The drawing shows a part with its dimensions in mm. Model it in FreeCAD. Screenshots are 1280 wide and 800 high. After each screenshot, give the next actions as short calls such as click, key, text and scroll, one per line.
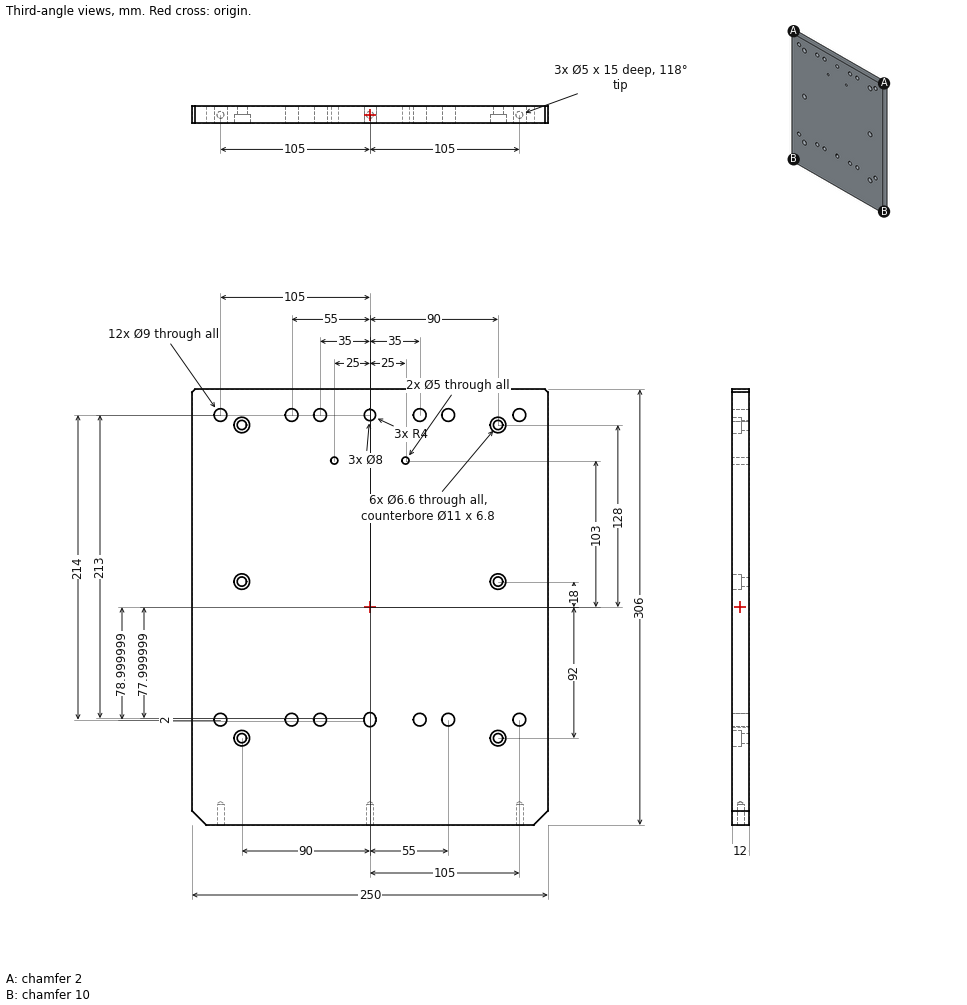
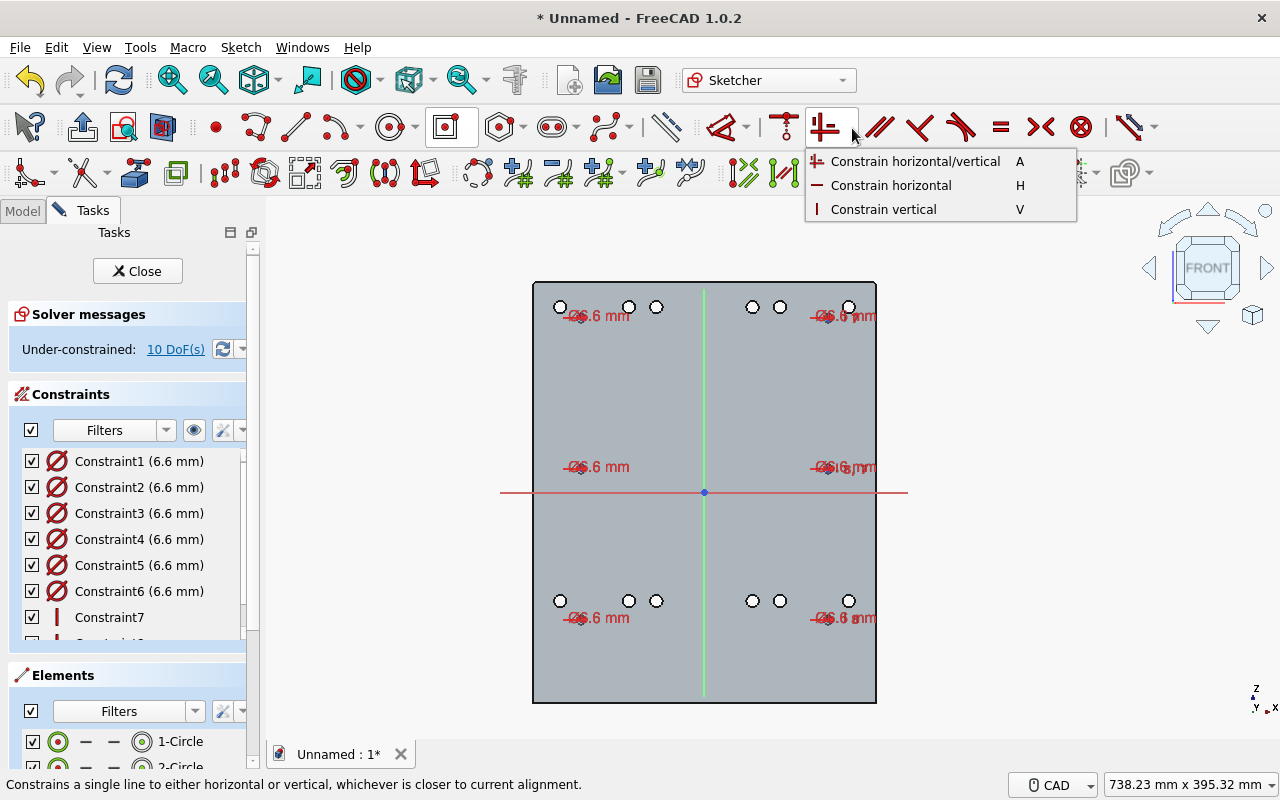
click(941, 185)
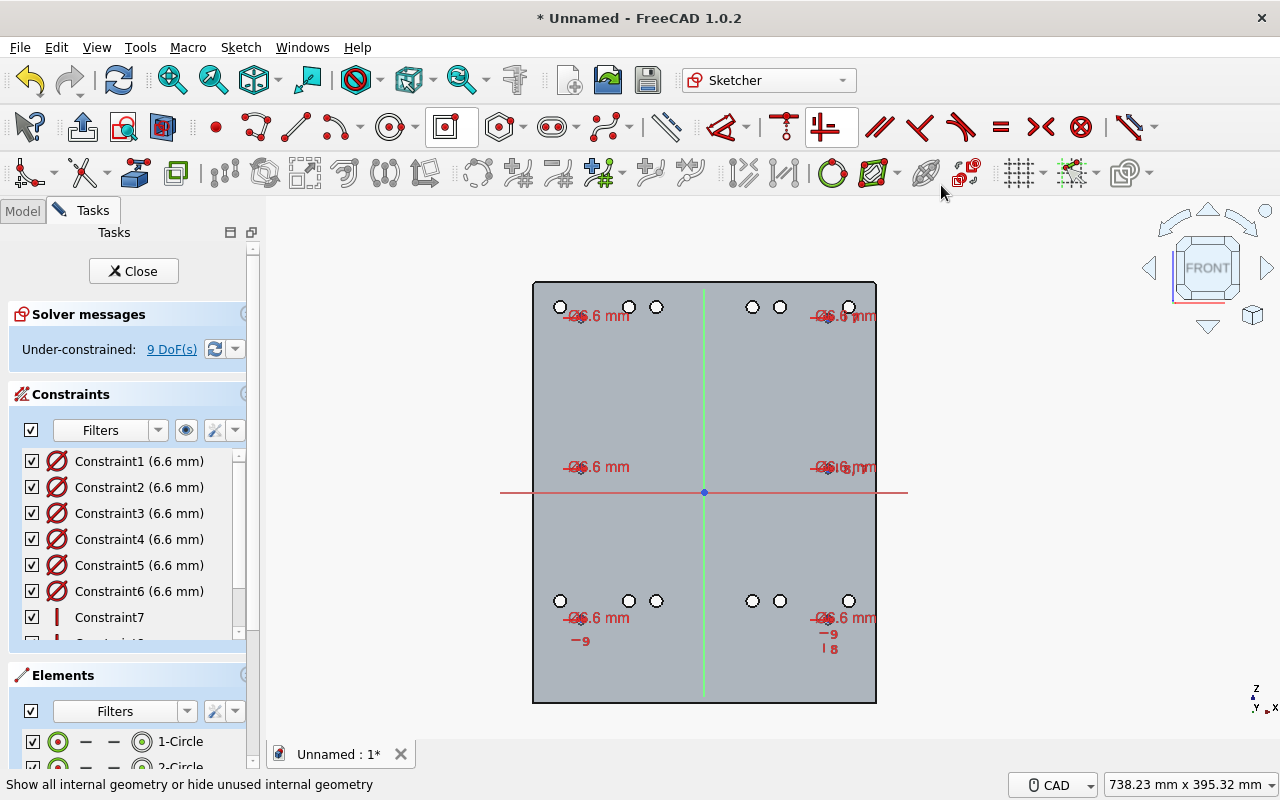
click(581, 620)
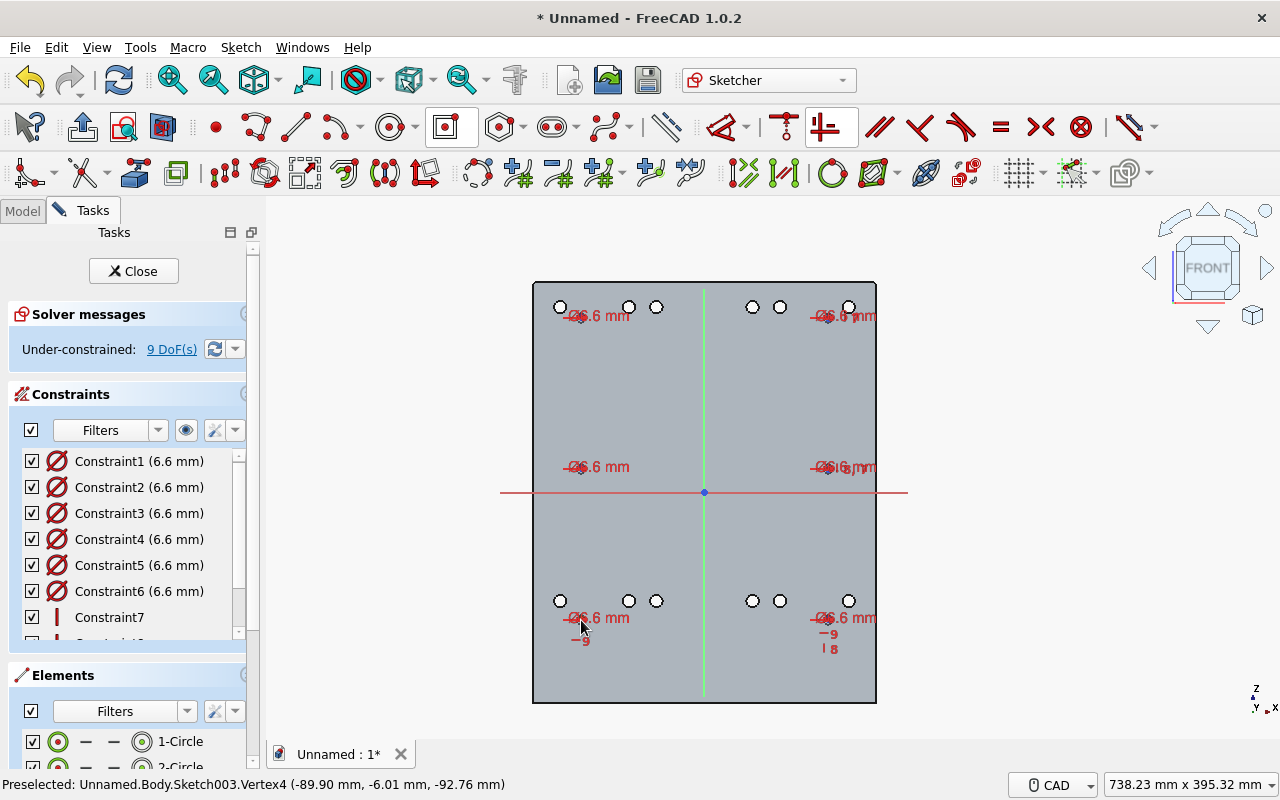
click(581, 469)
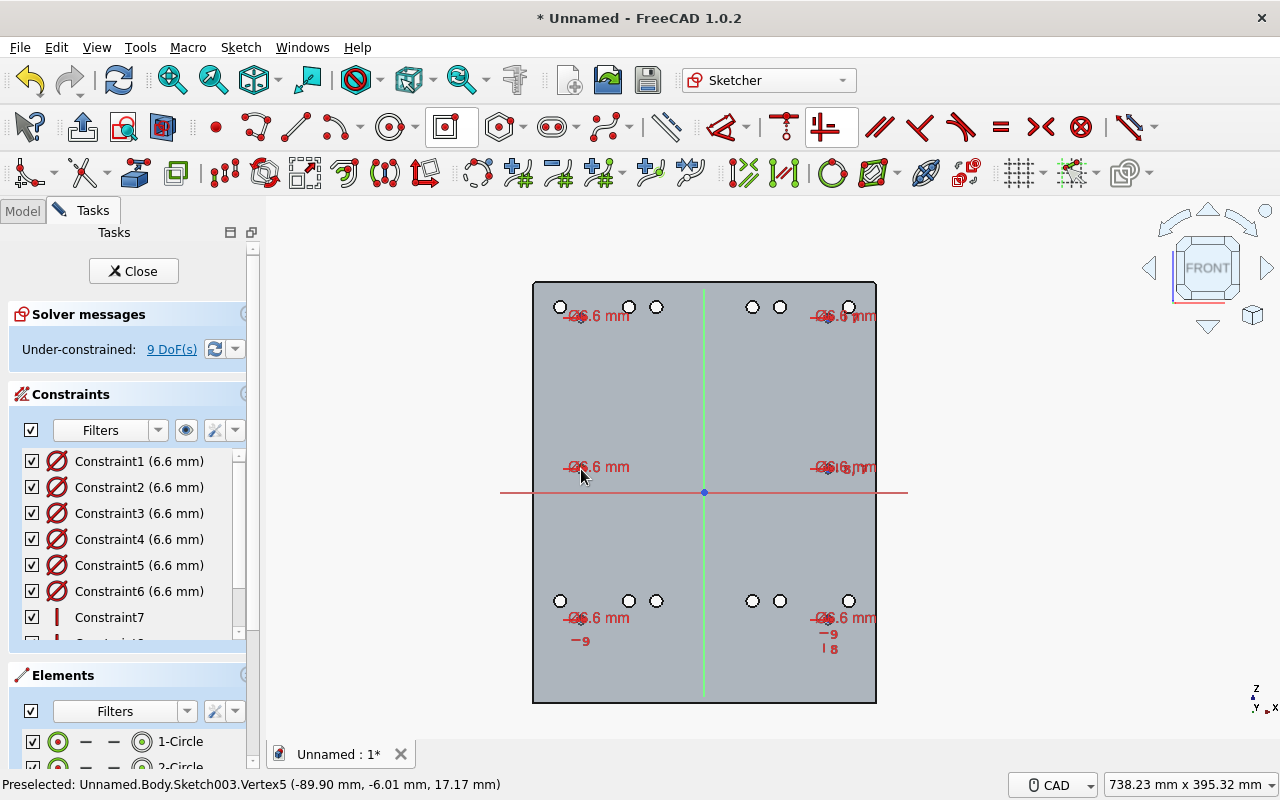
click(852, 128)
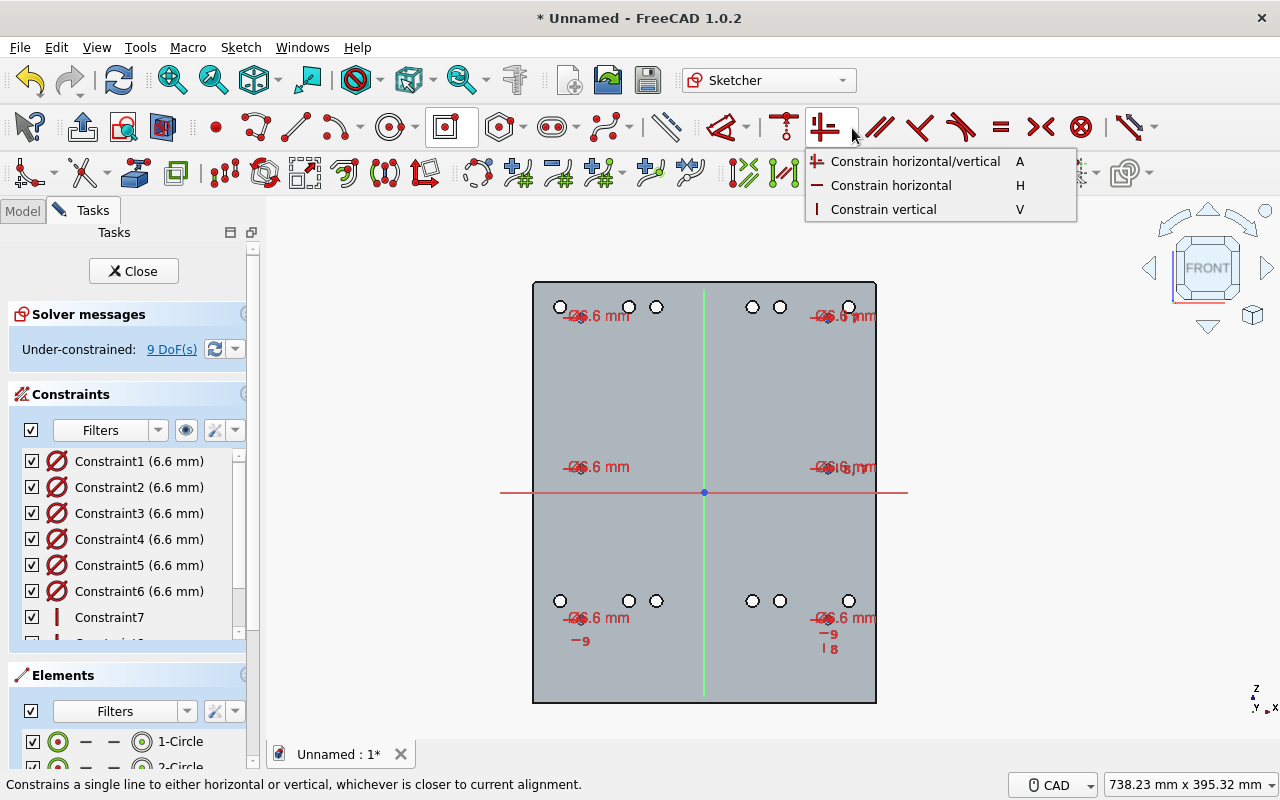
click(941, 209)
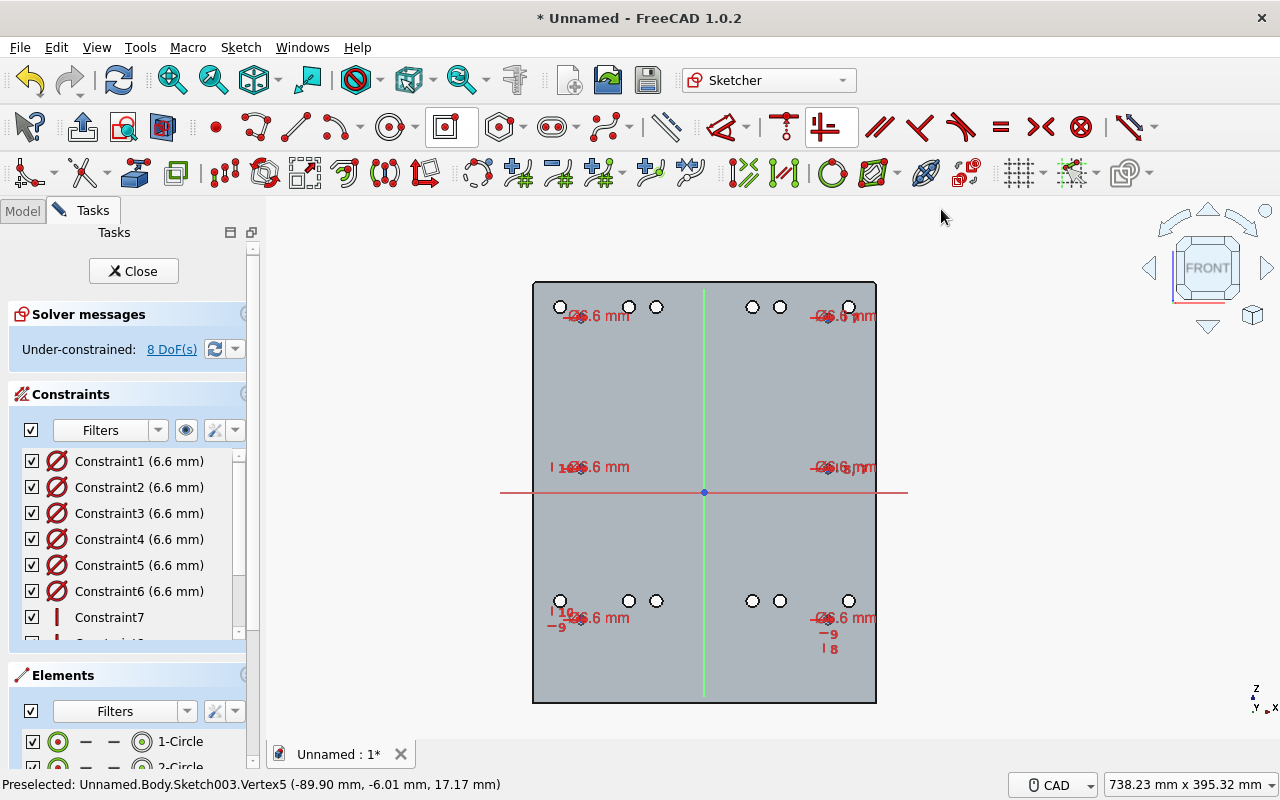
click(828, 469)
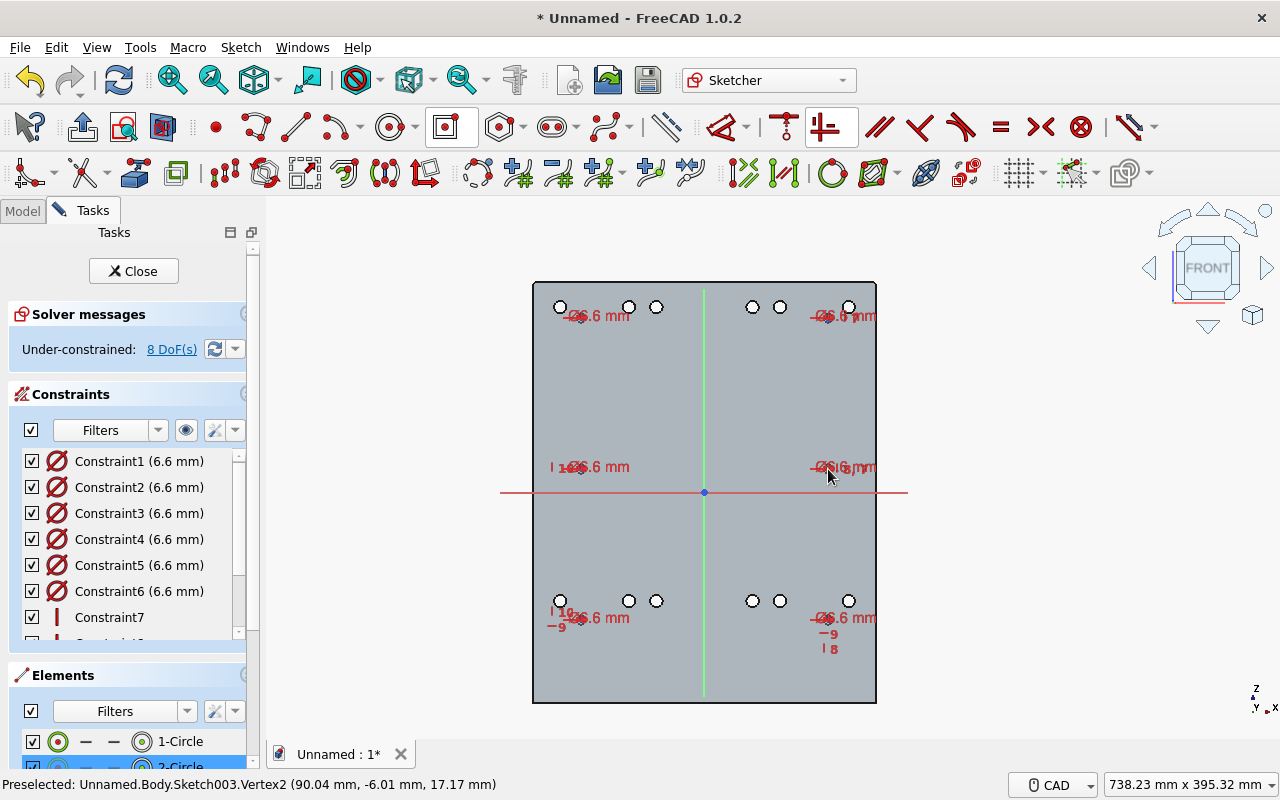
click(581, 469)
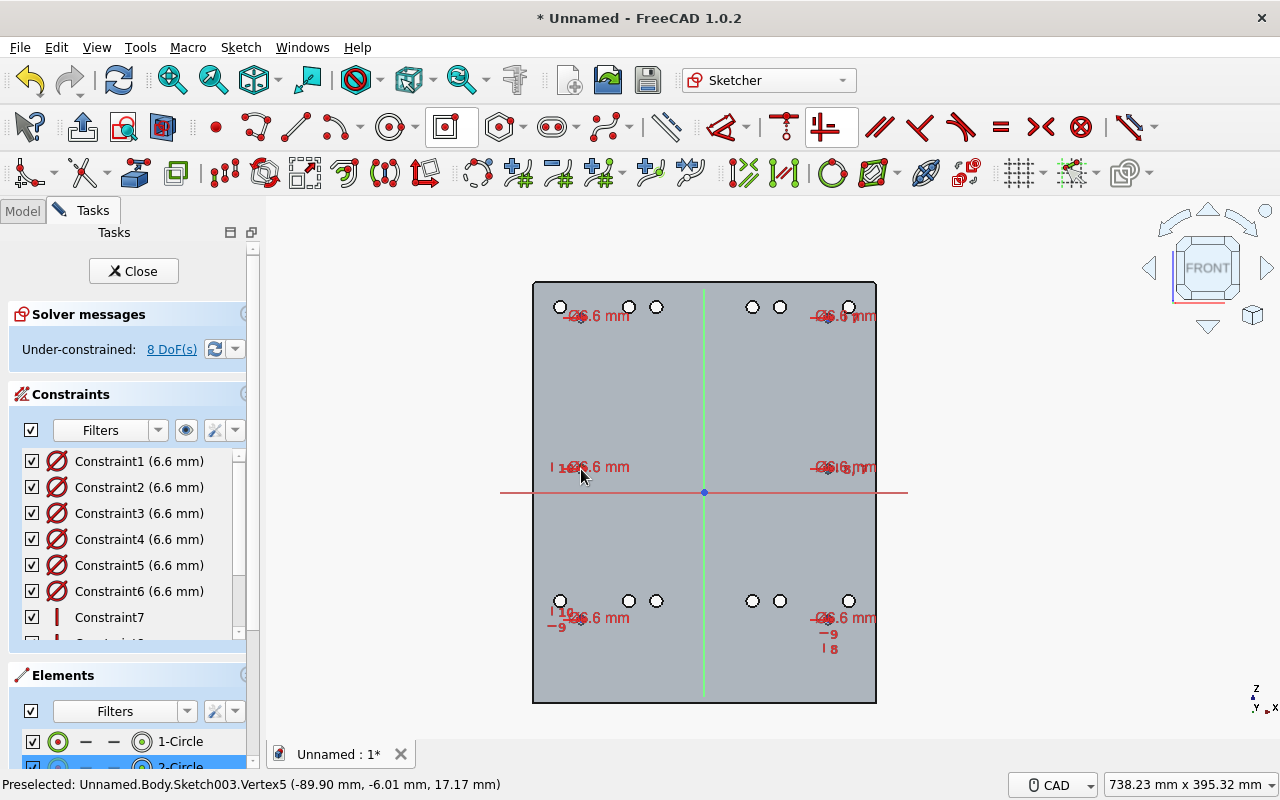
key(h)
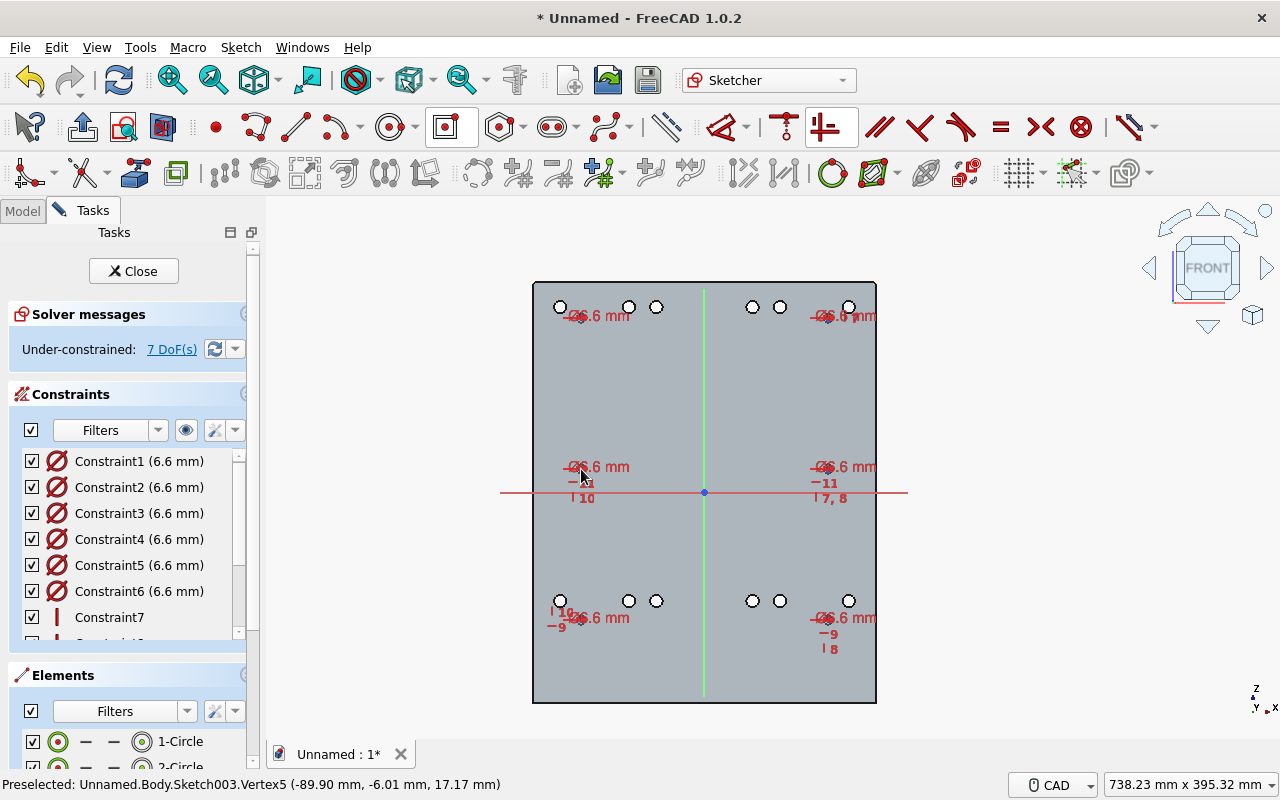
click(581, 469)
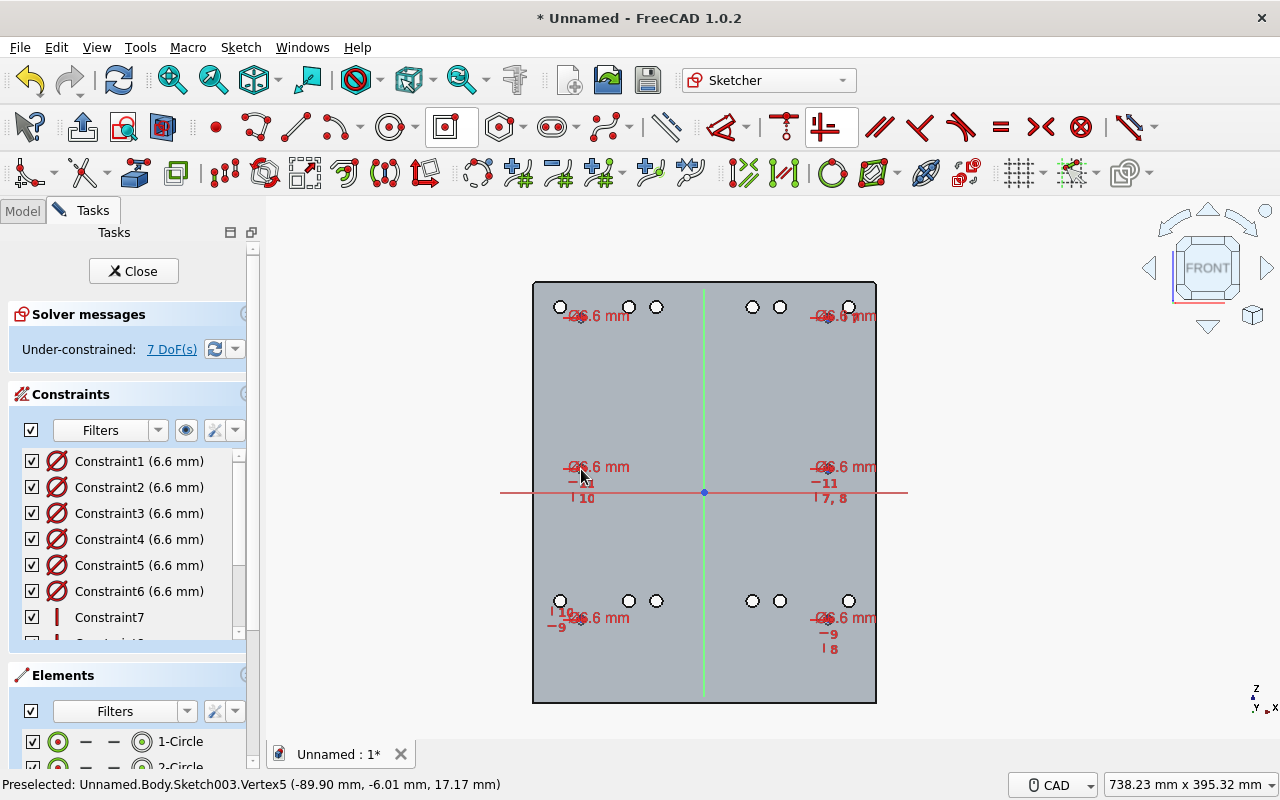
click(581, 318)